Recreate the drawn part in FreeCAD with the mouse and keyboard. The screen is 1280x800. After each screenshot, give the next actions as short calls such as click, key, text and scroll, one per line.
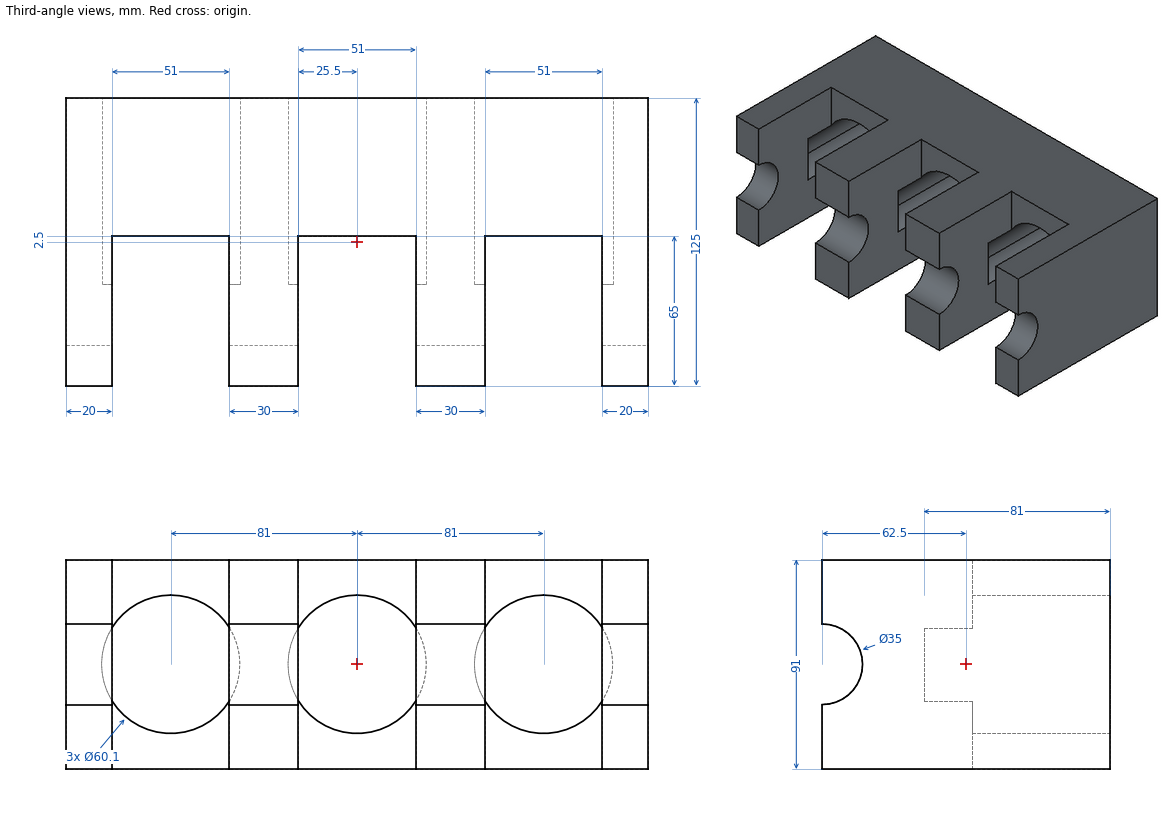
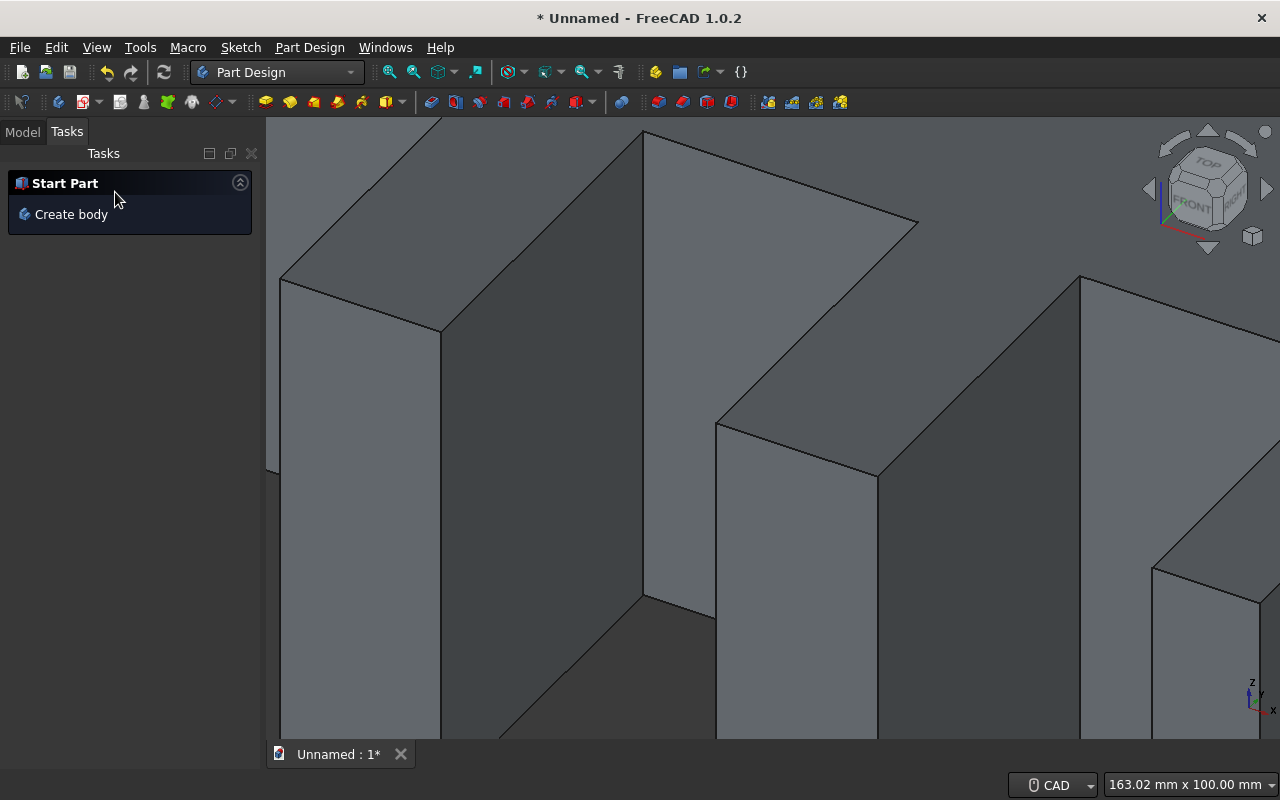
click(390, 72)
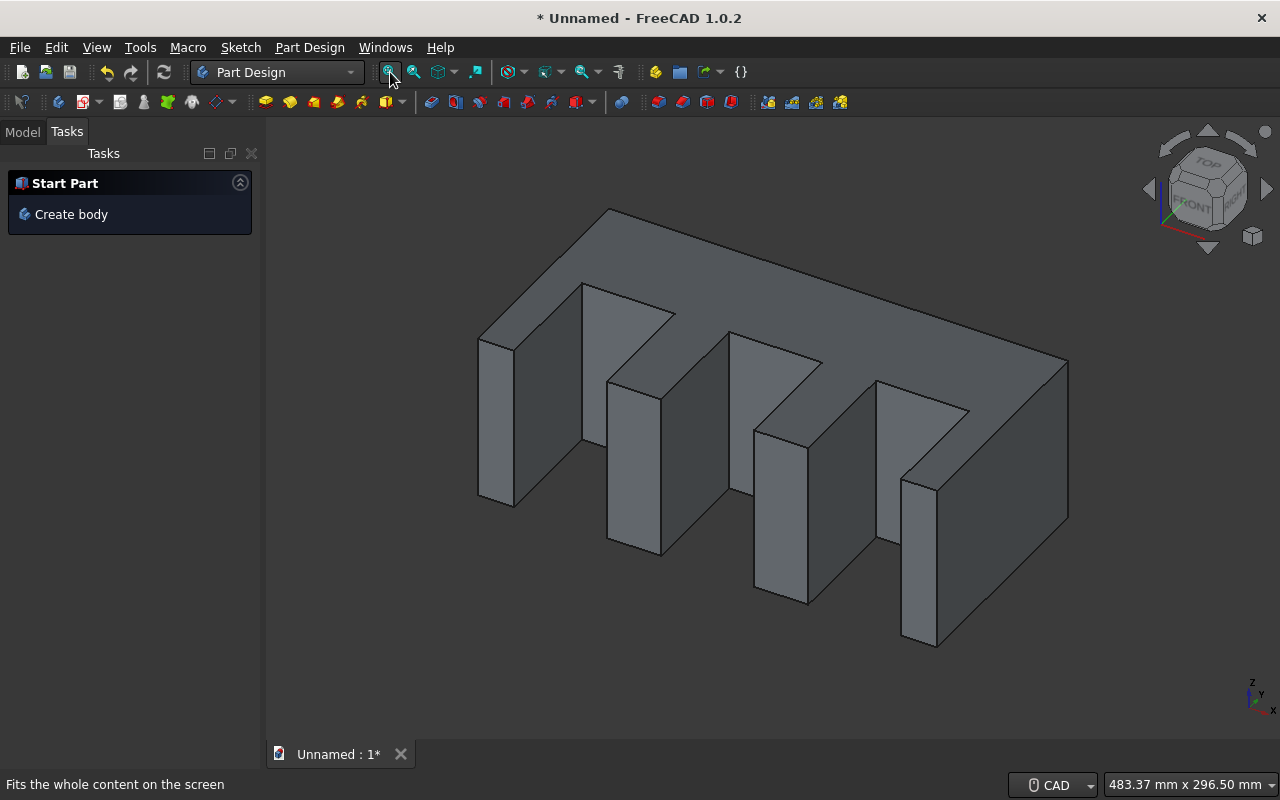
click(1003, 503)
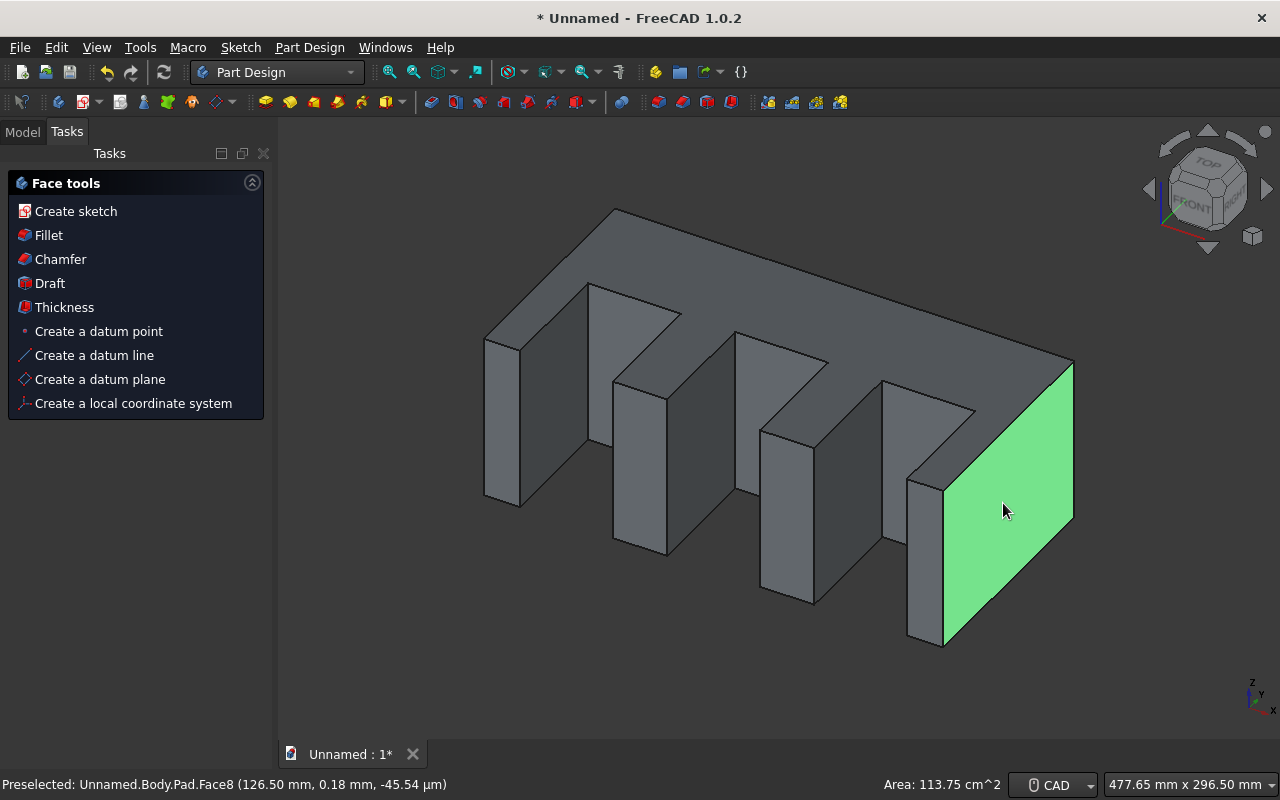
click(84, 102)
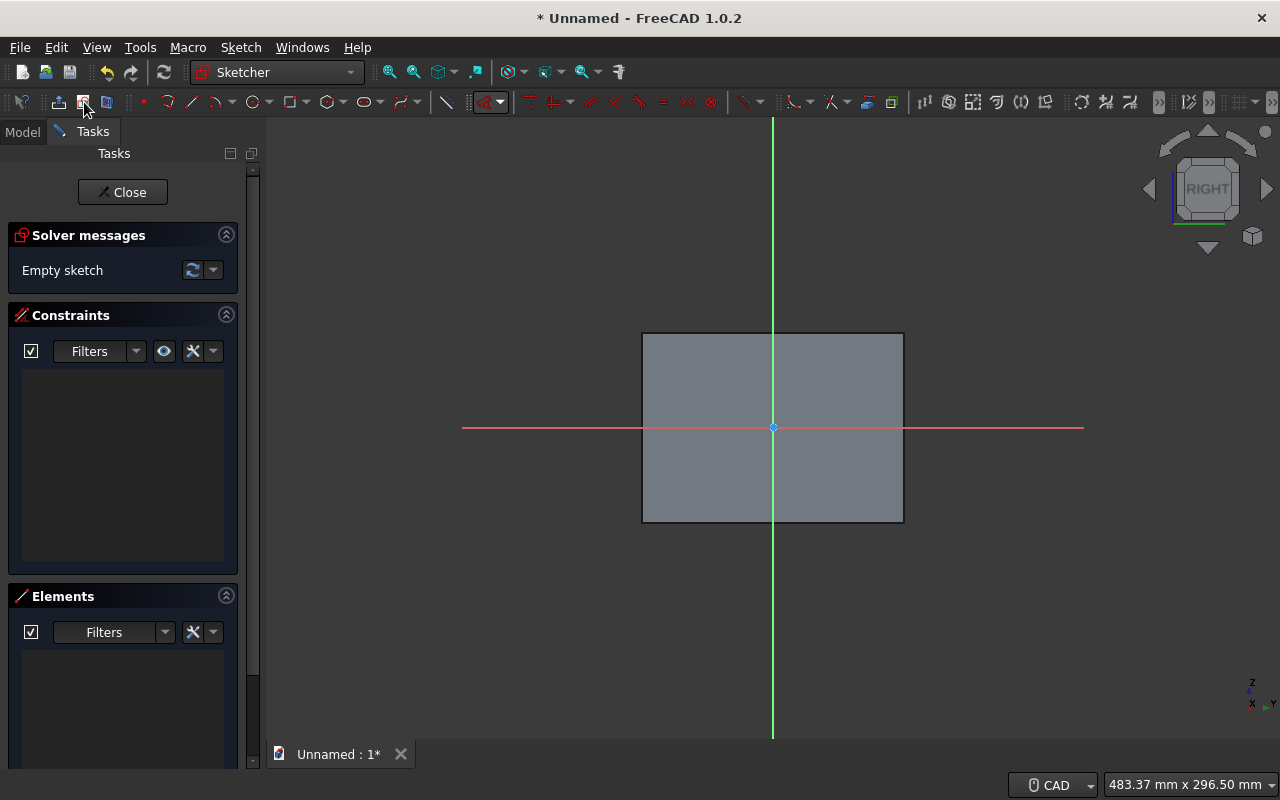
scroll(682, 428, up, 6)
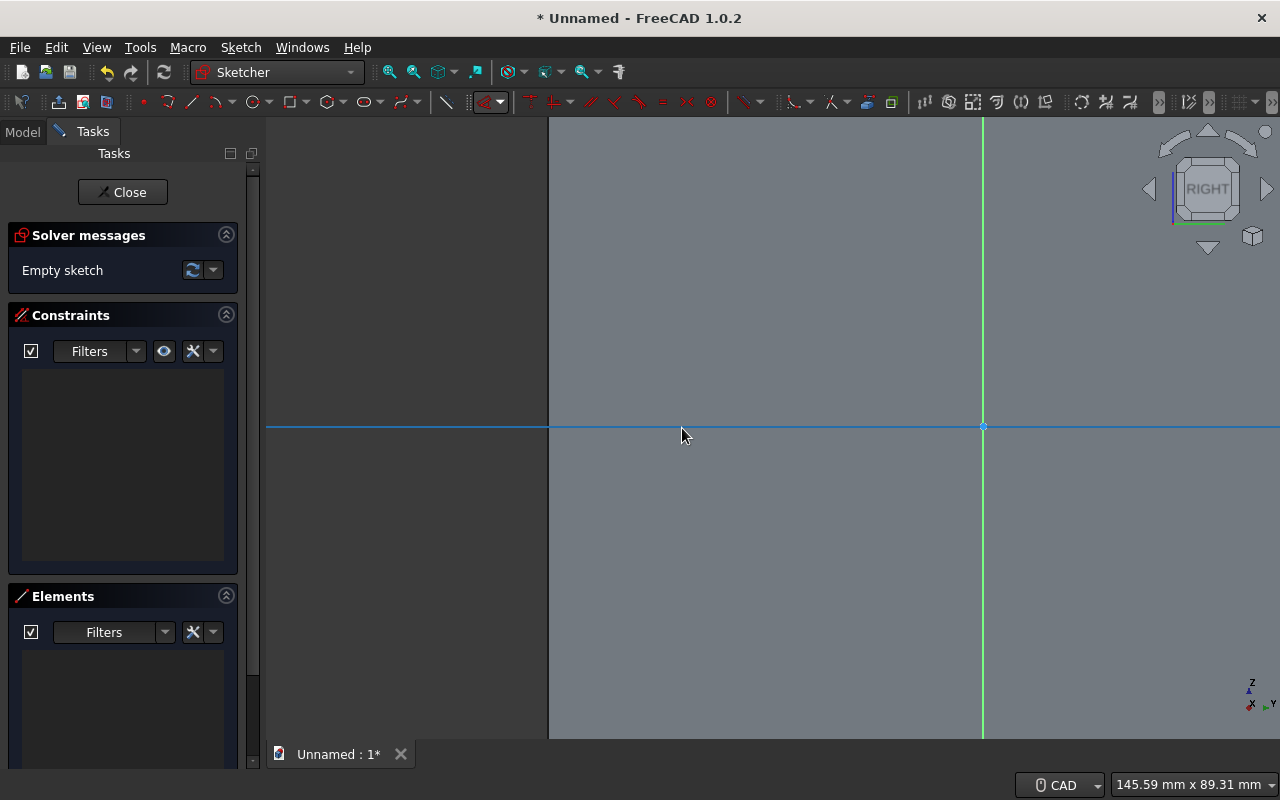
key(g)
key(c)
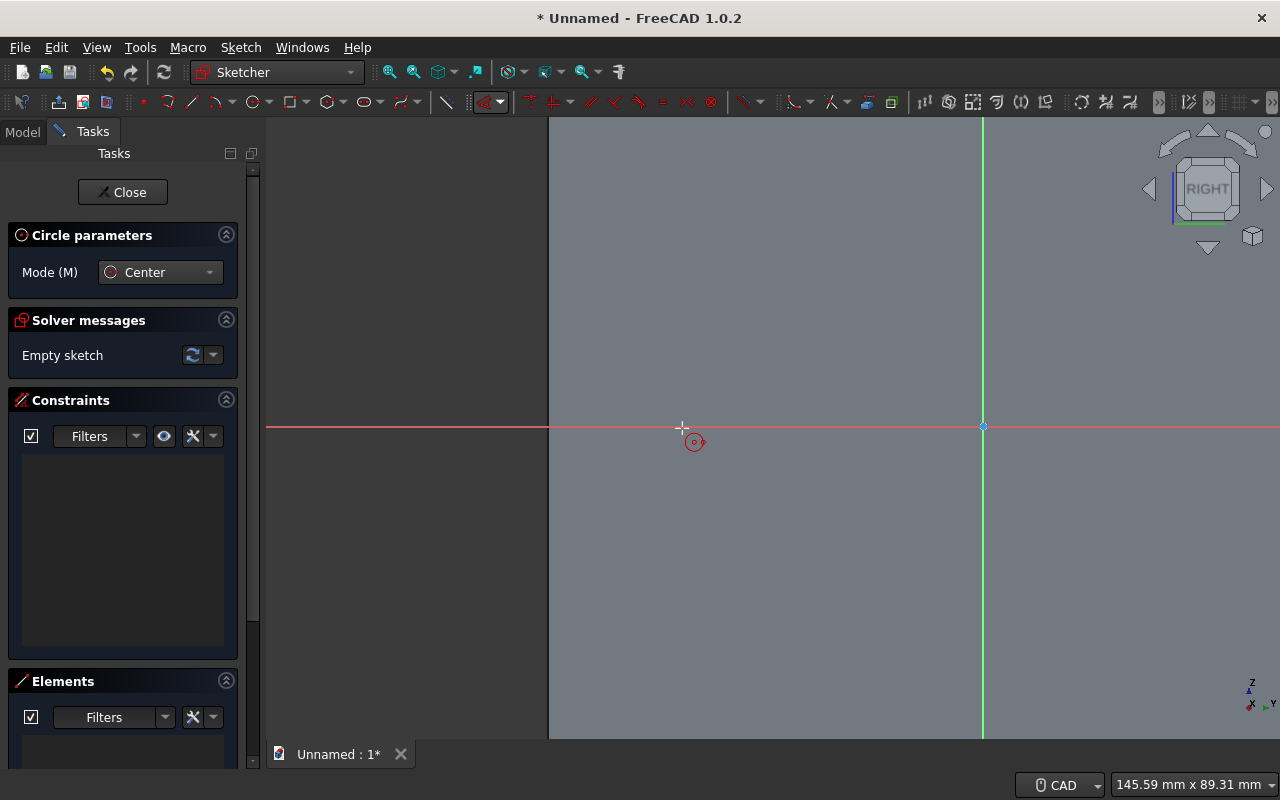
click(548, 427)
move(634, 341)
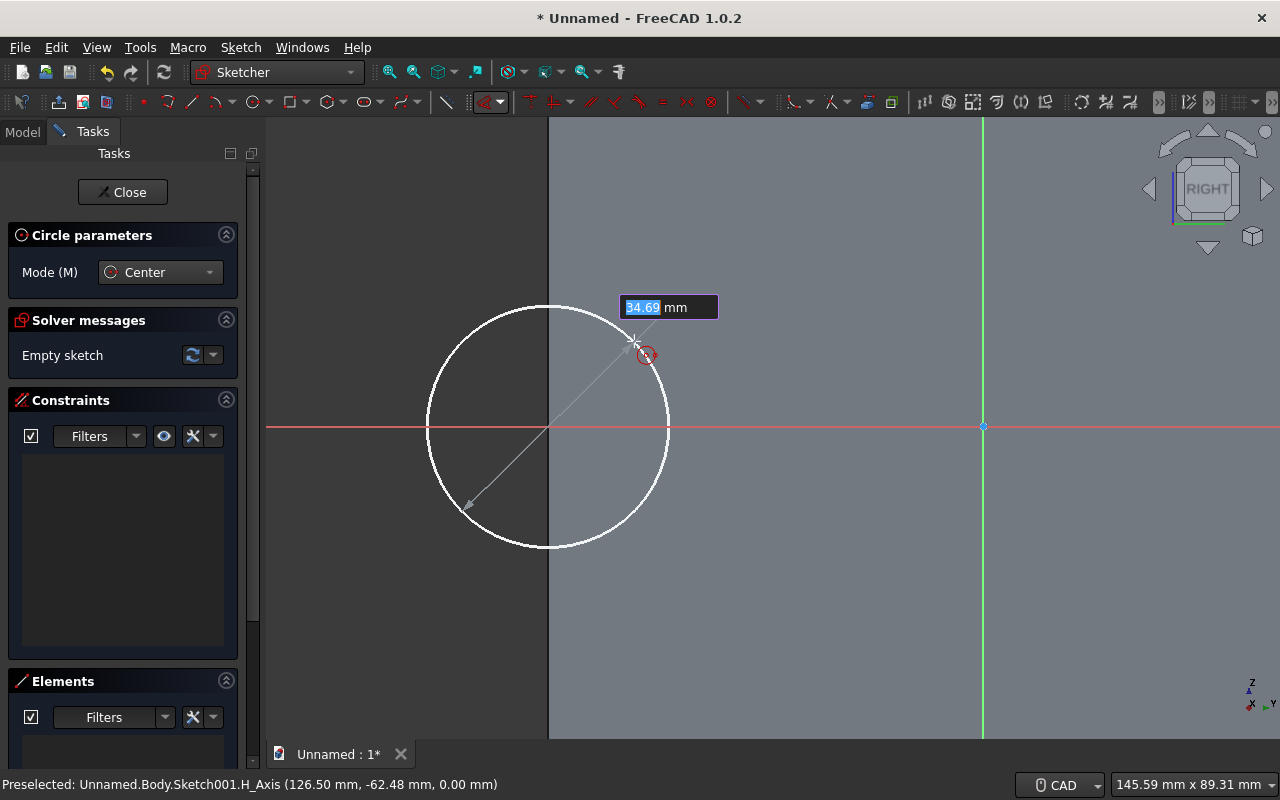
text(35)
key(Return)
key(Escape)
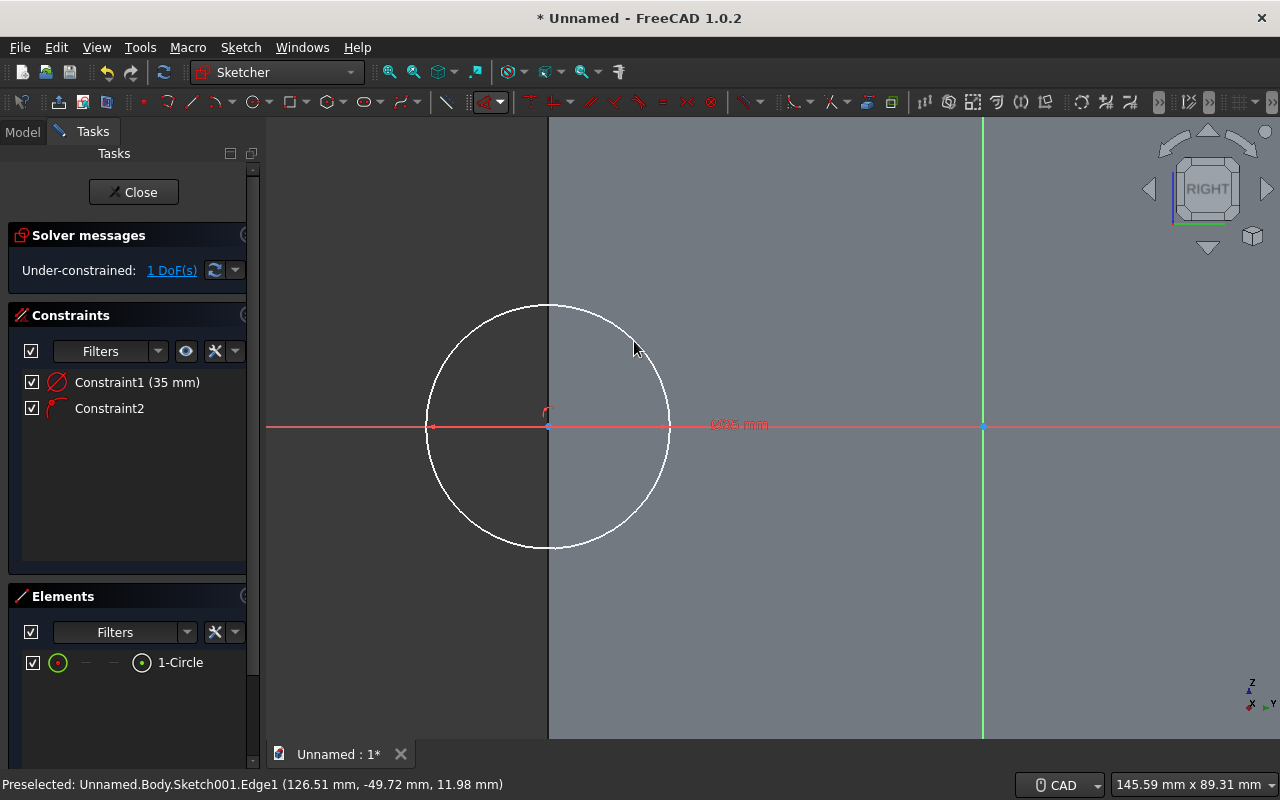
click(548, 427)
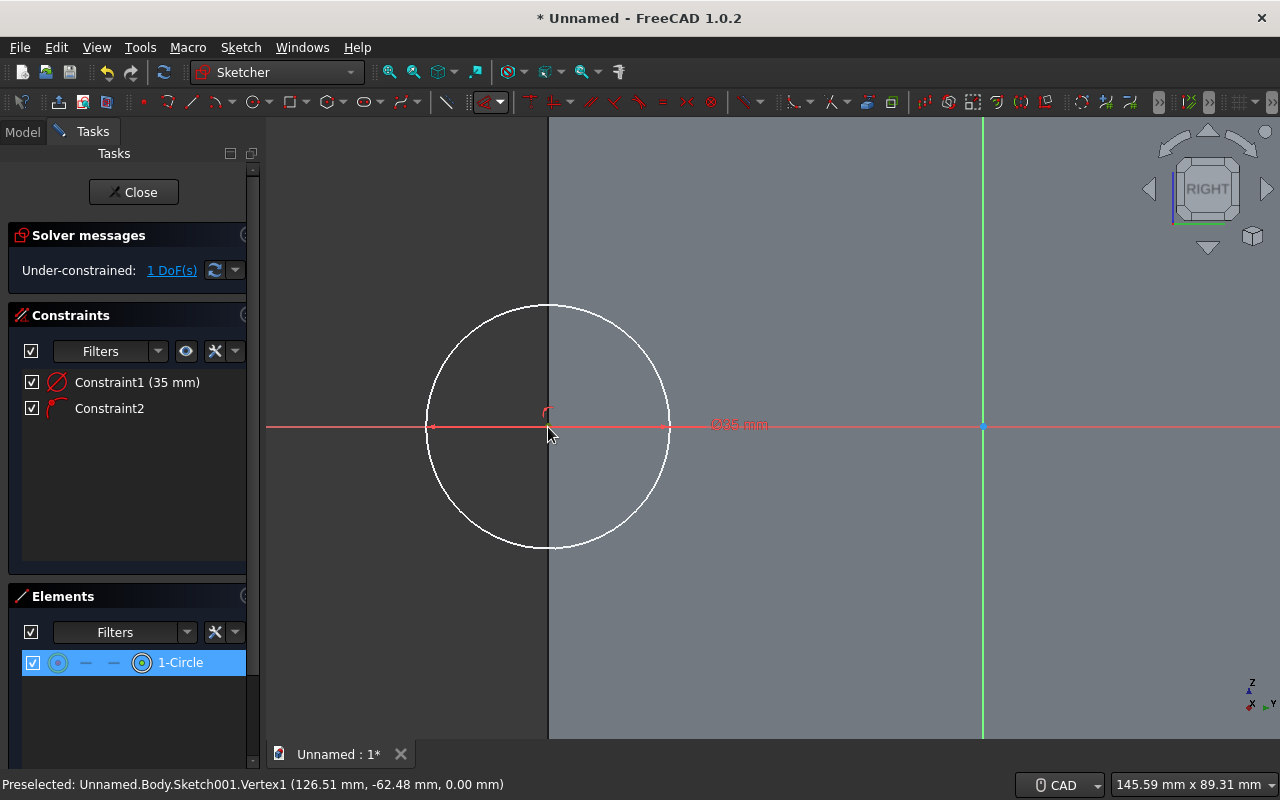
key(l)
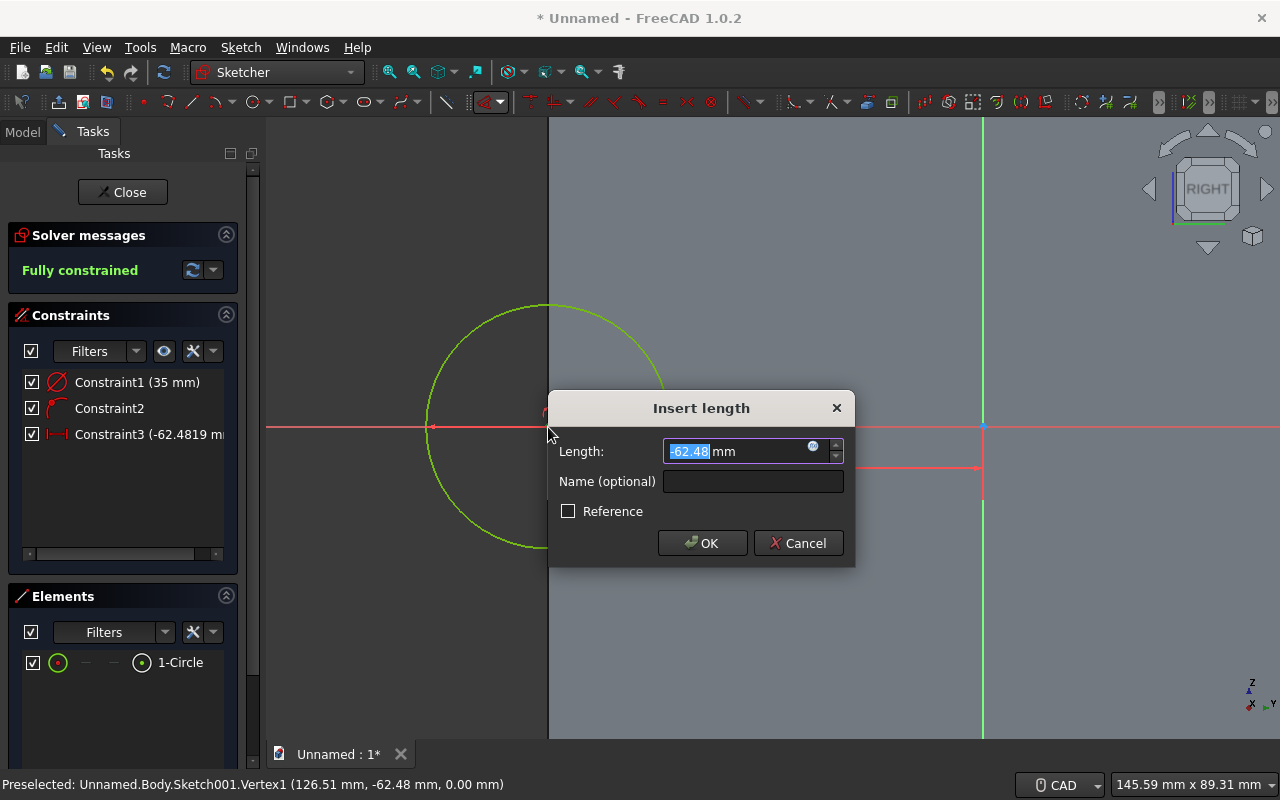
text(-62.5)
key(Return)